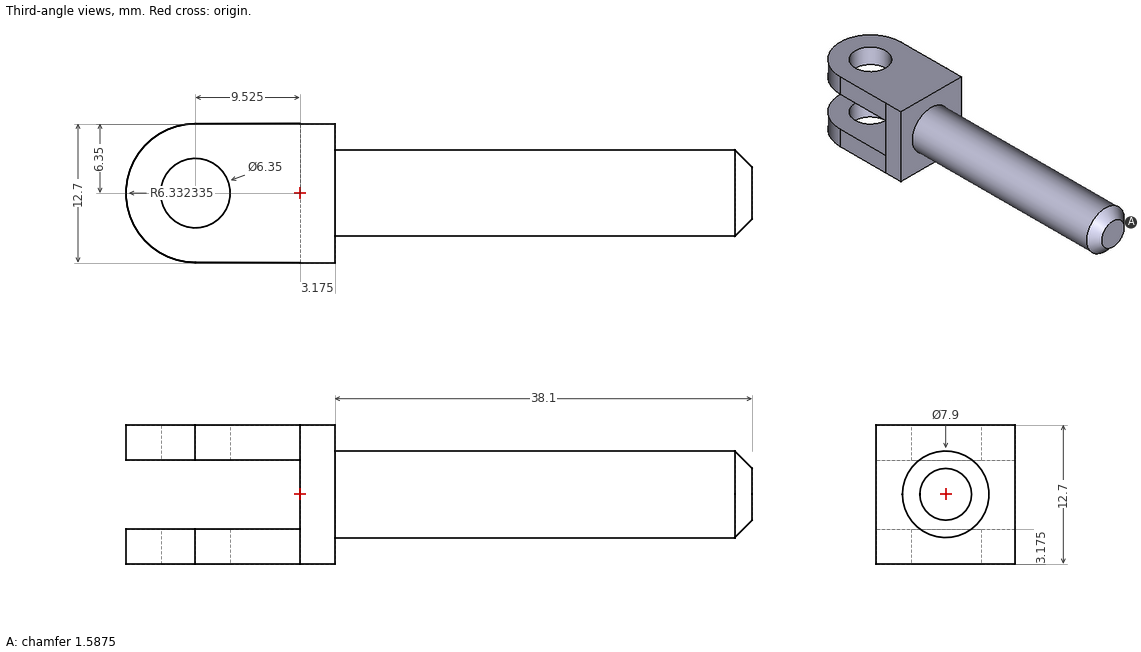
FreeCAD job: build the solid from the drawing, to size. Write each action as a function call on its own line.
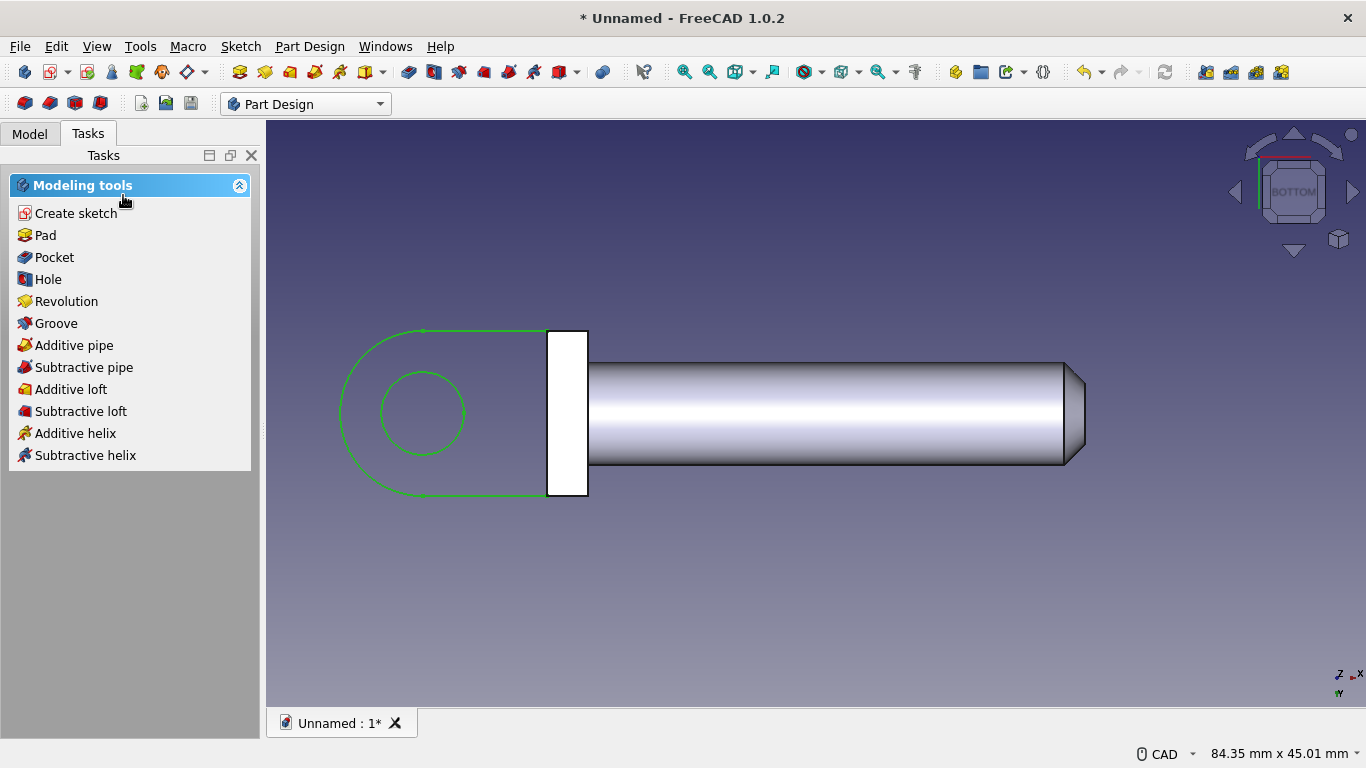
click(240, 72)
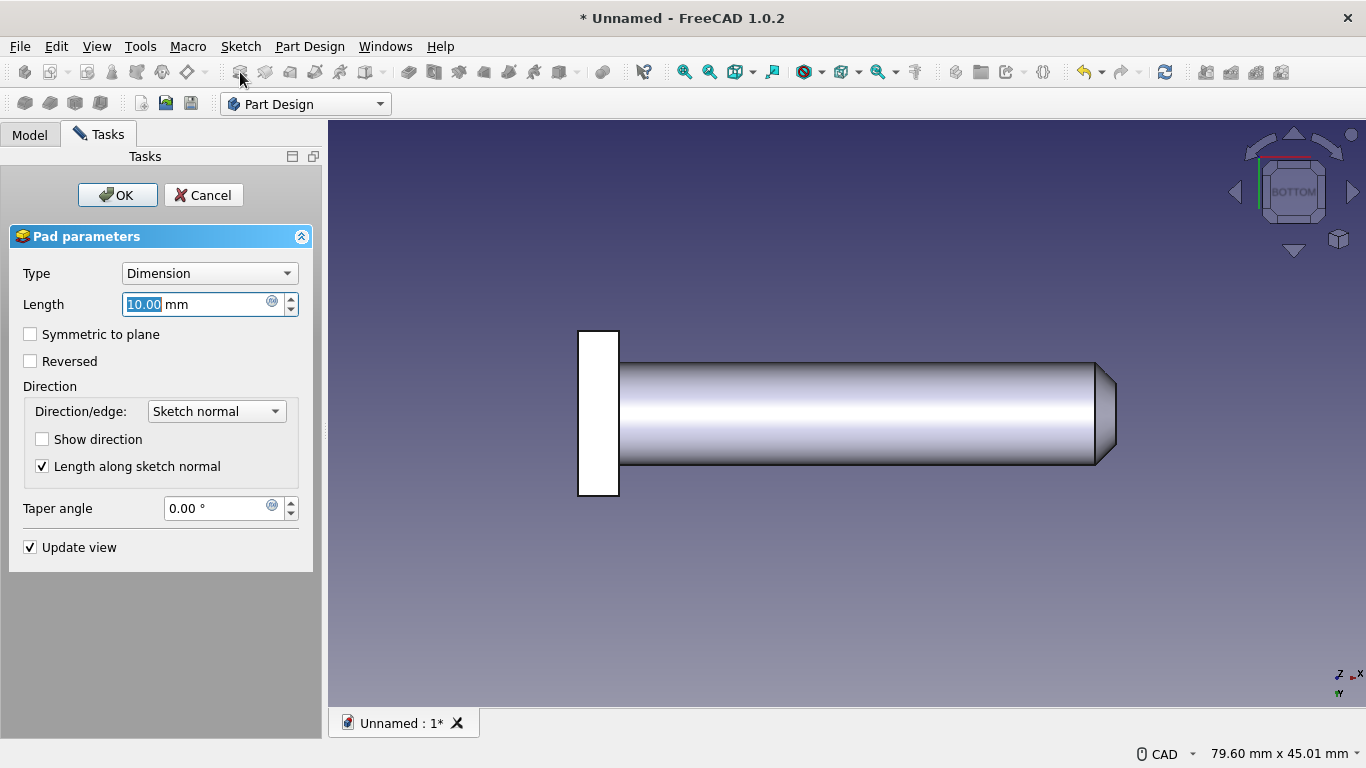
text(3.175)
key(Tab)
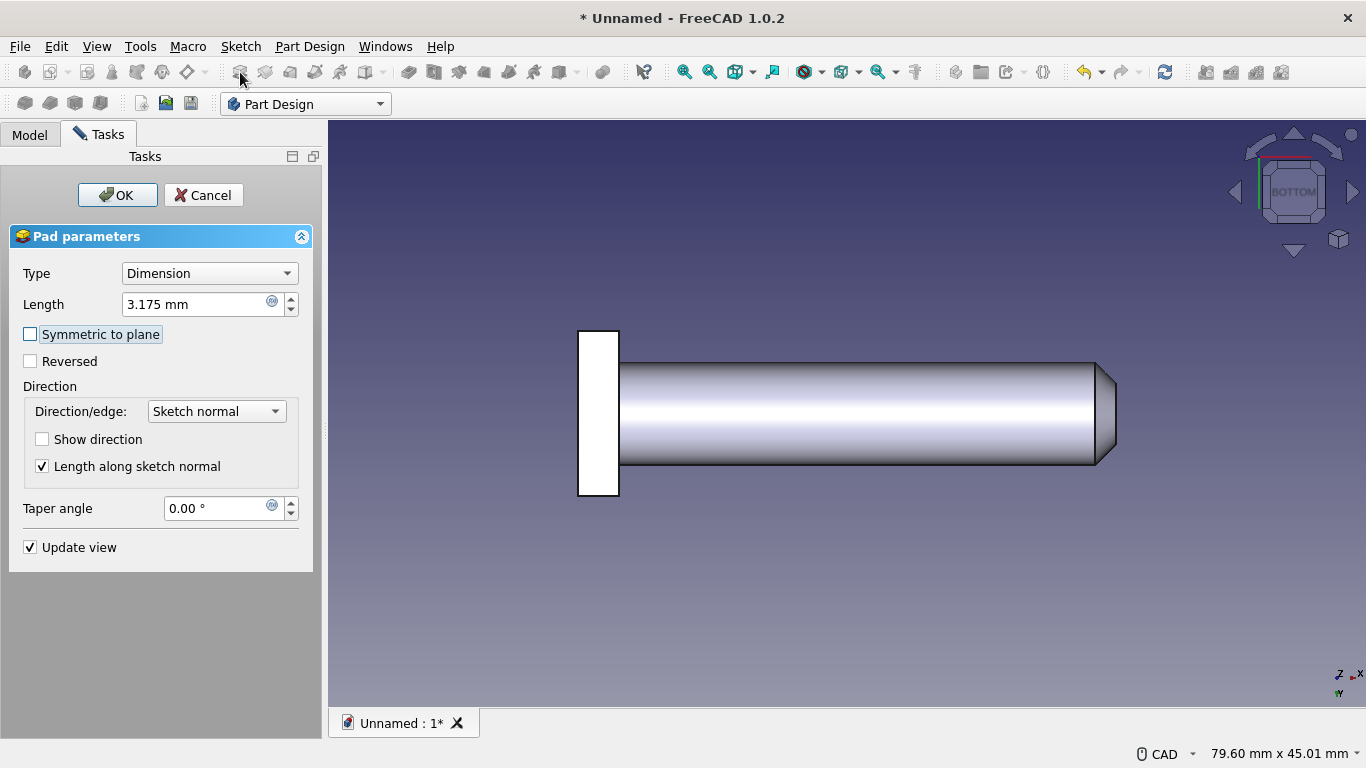
click(31, 361)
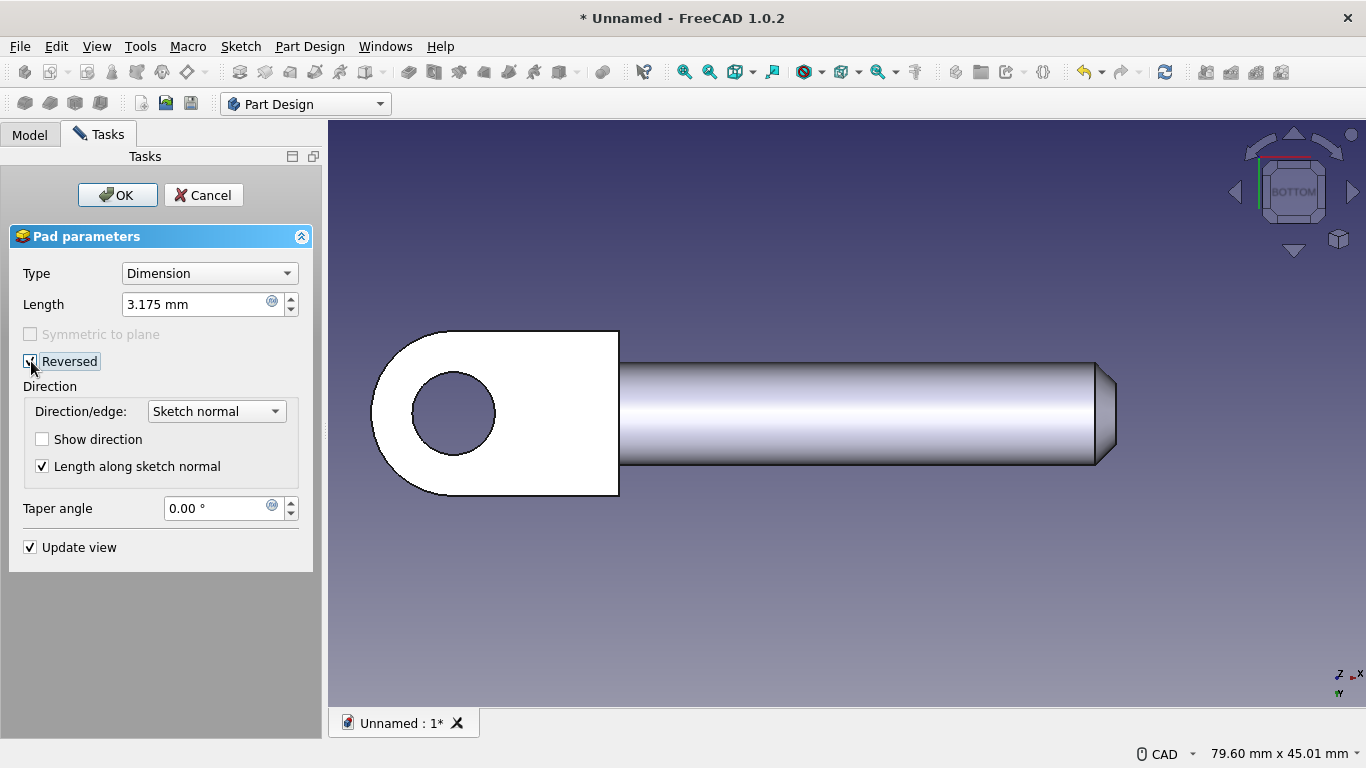
click(118, 195)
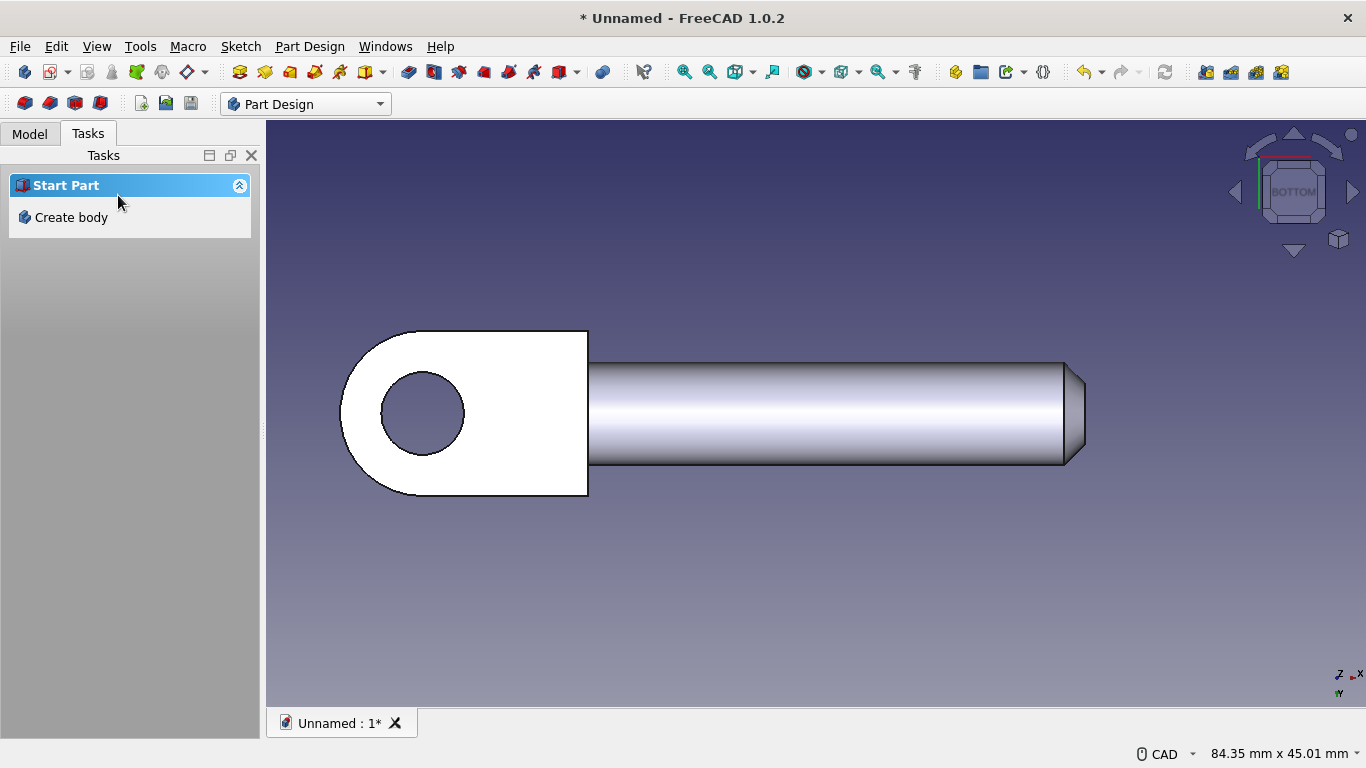
click(30, 134)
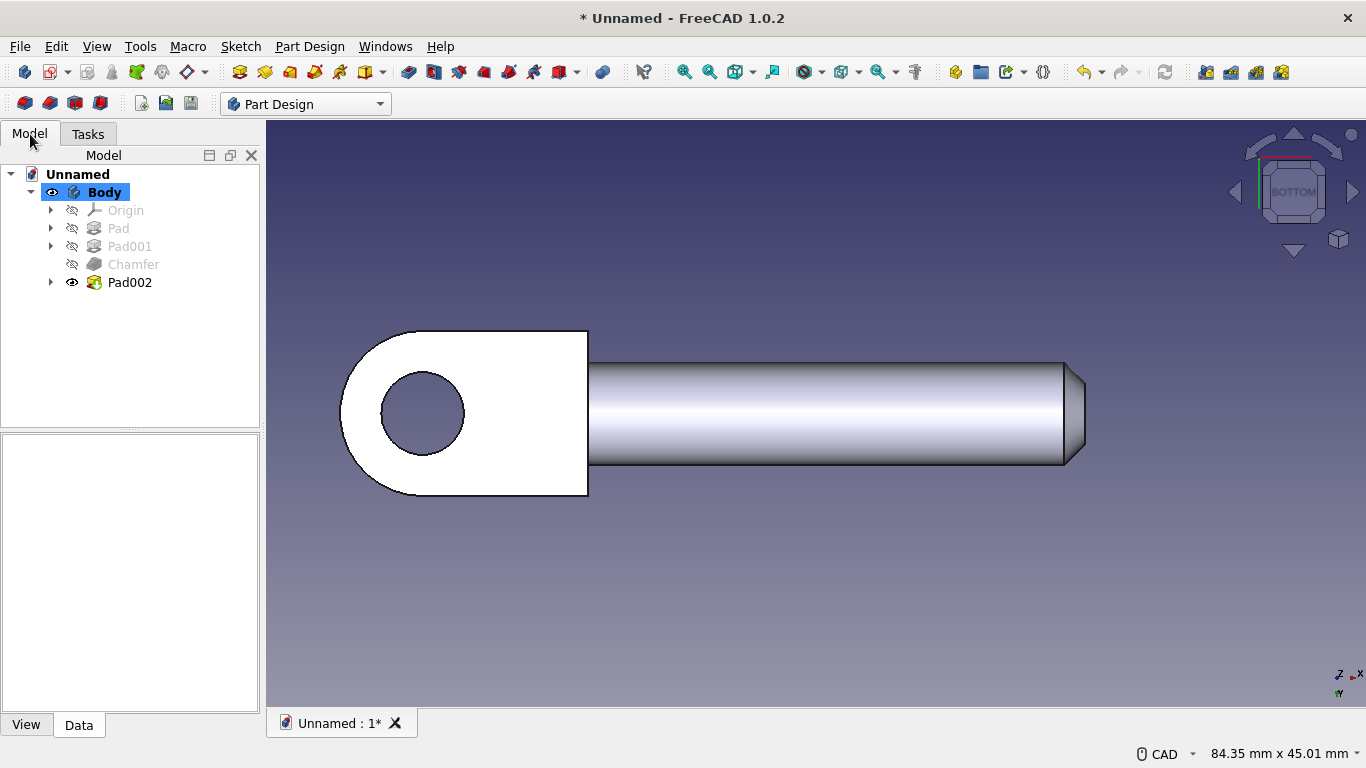
click(117, 282)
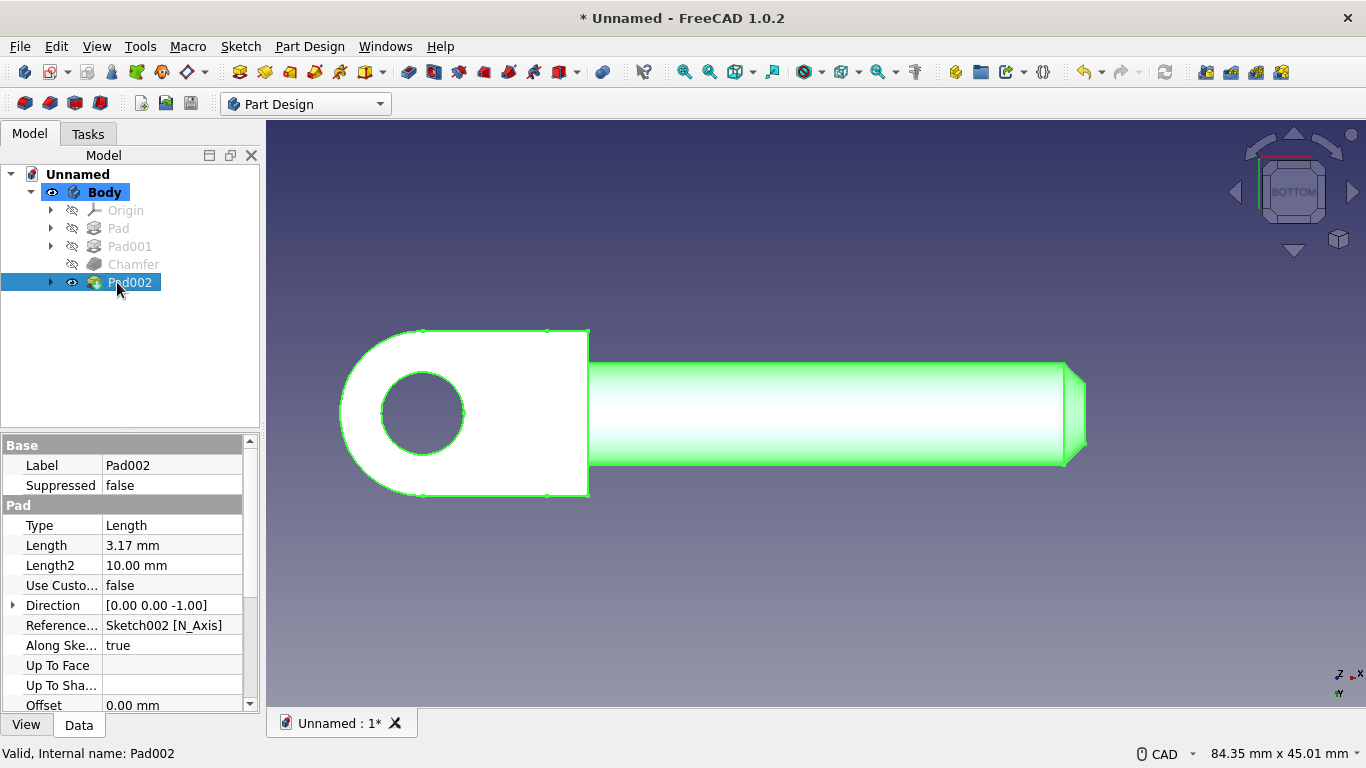
click(1206, 72)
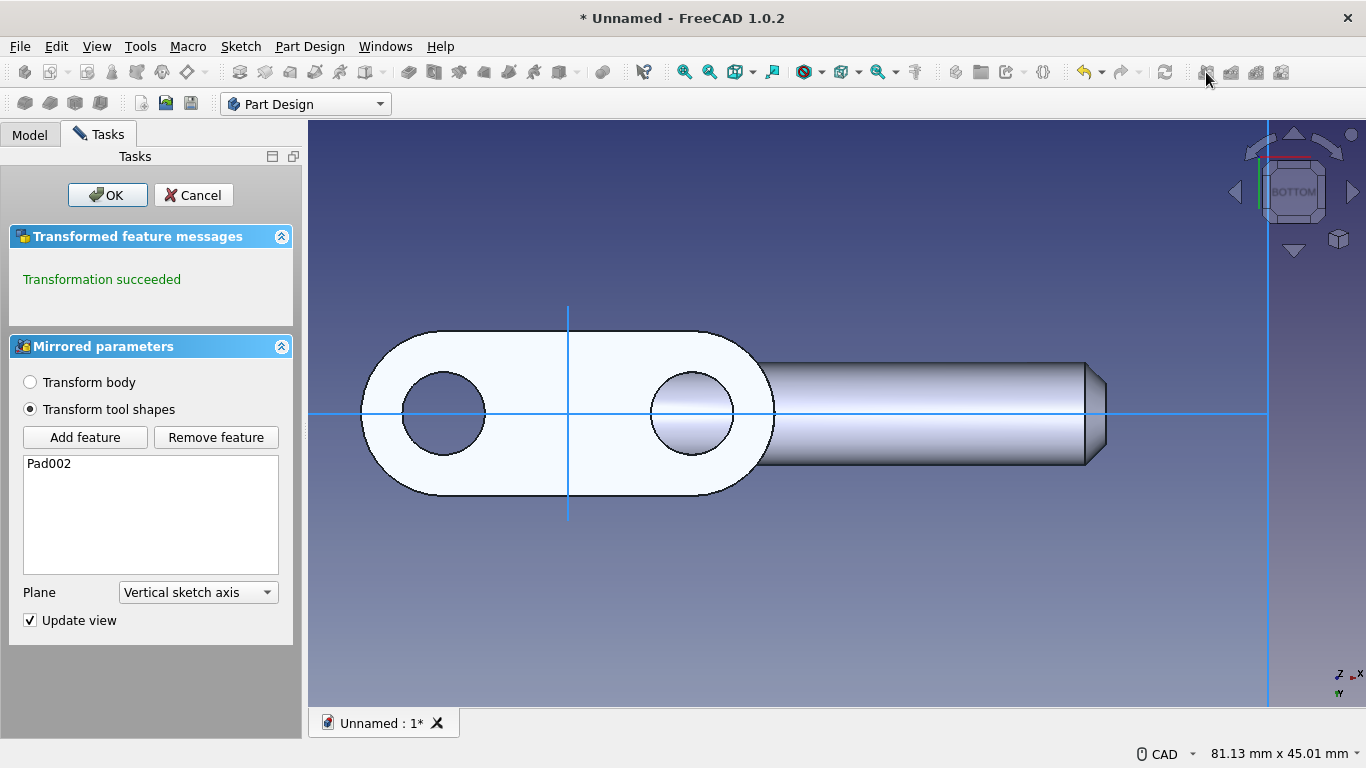
click(199, 592)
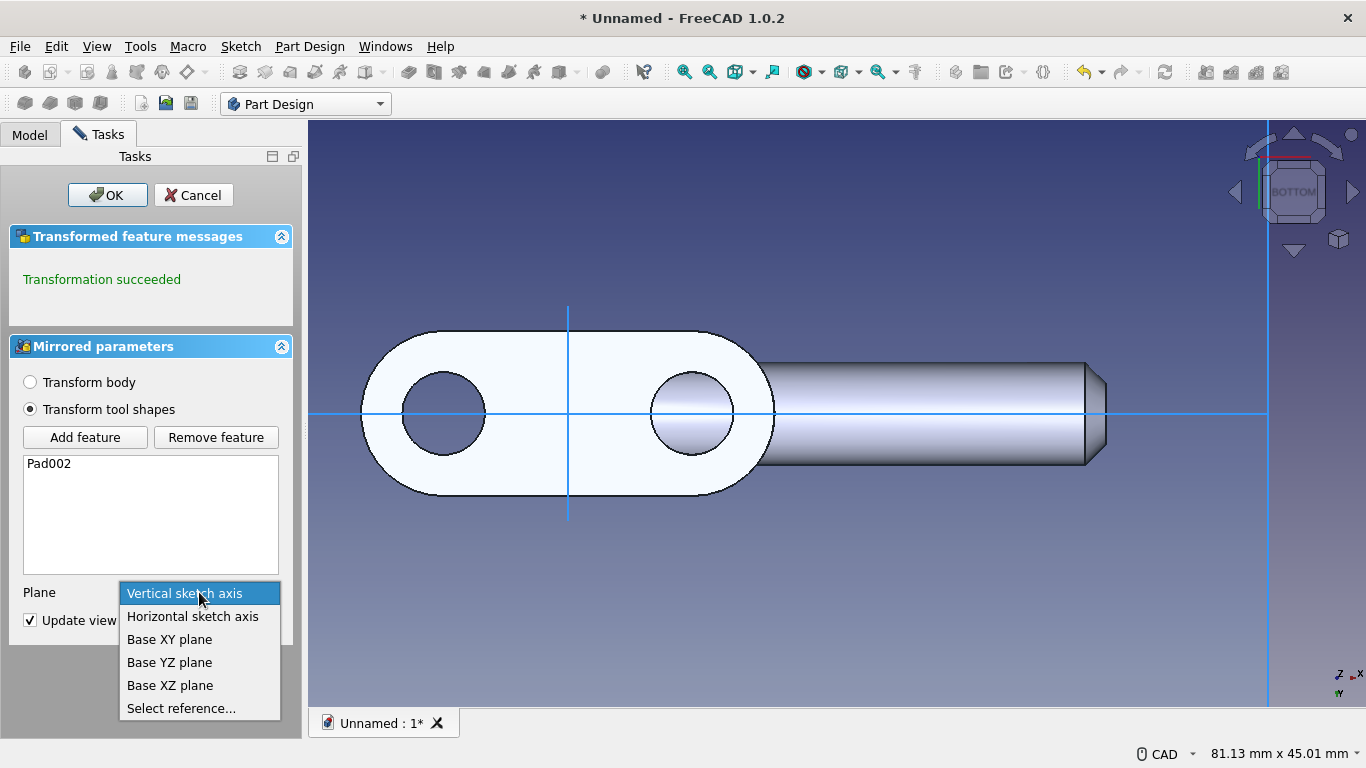
click(198, 640)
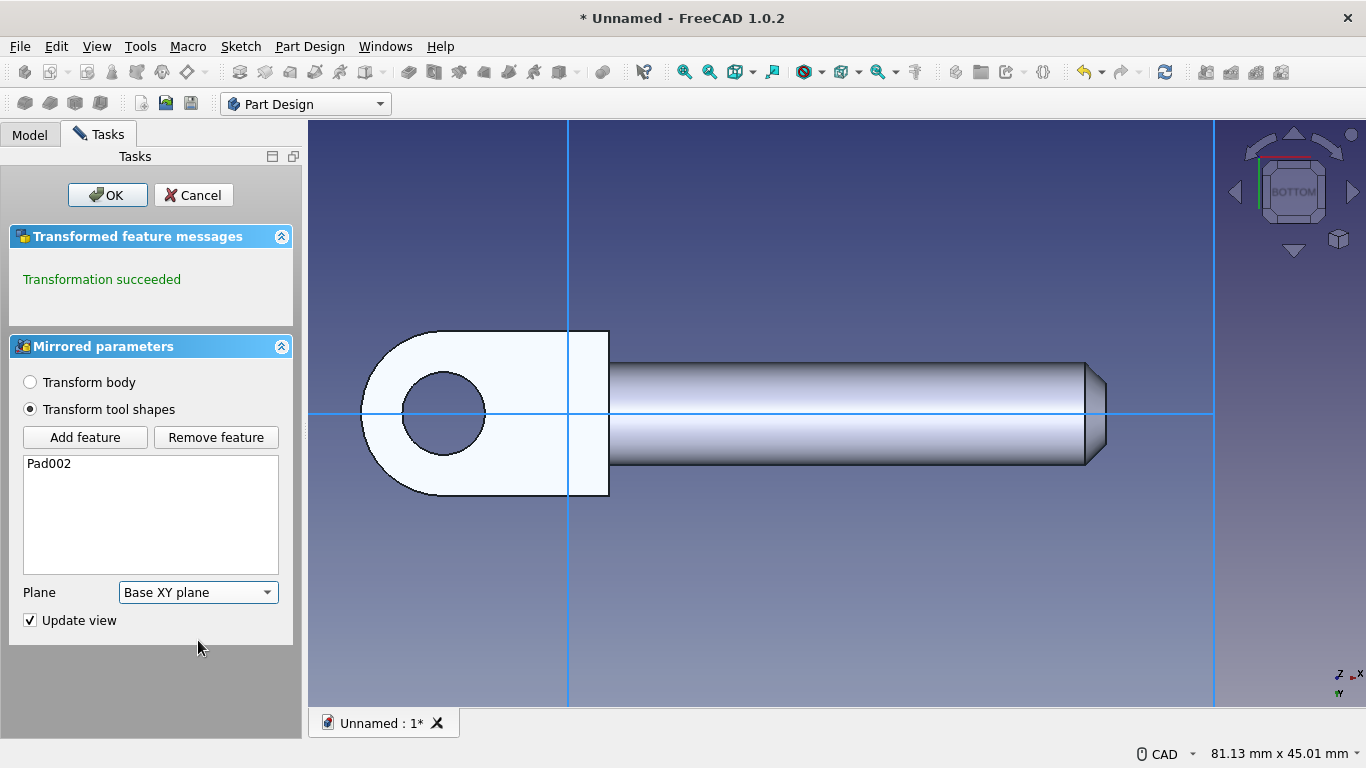
click(108, 195)